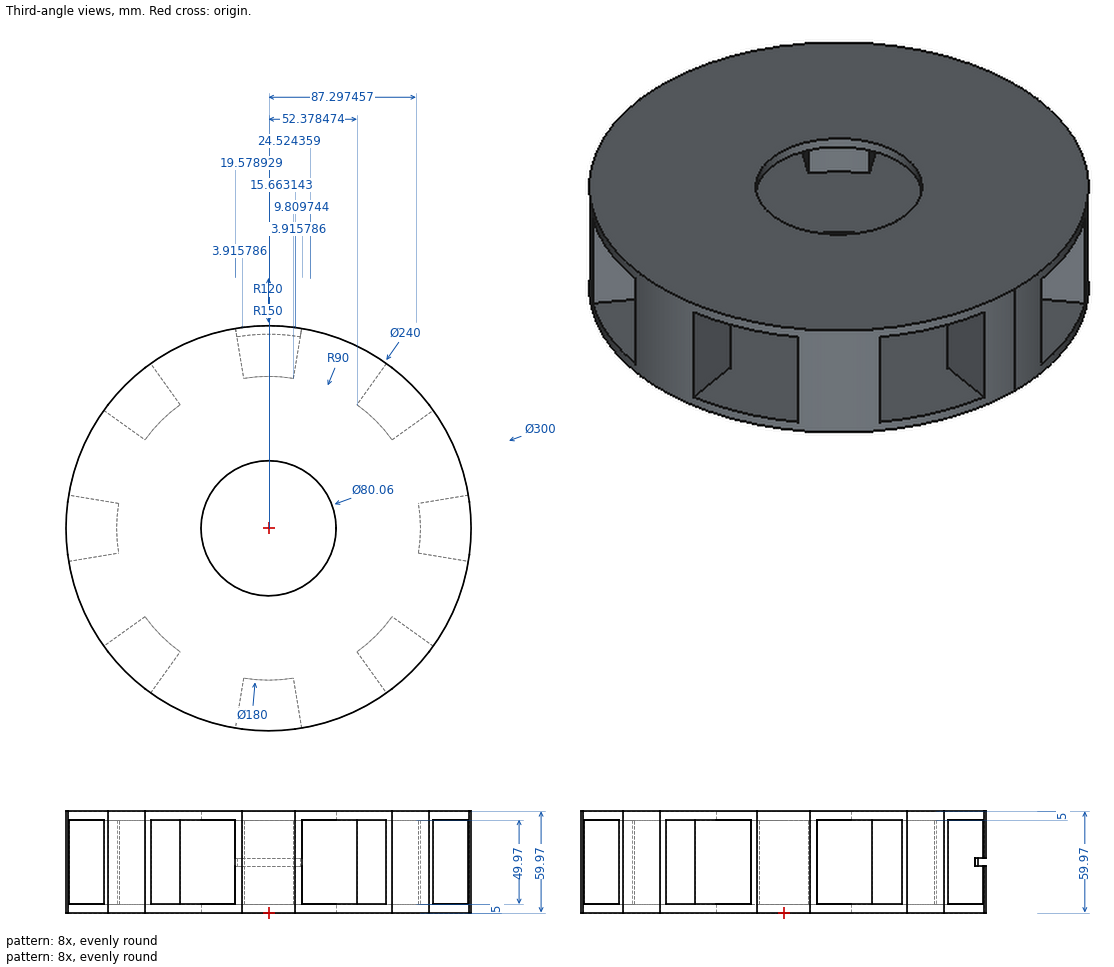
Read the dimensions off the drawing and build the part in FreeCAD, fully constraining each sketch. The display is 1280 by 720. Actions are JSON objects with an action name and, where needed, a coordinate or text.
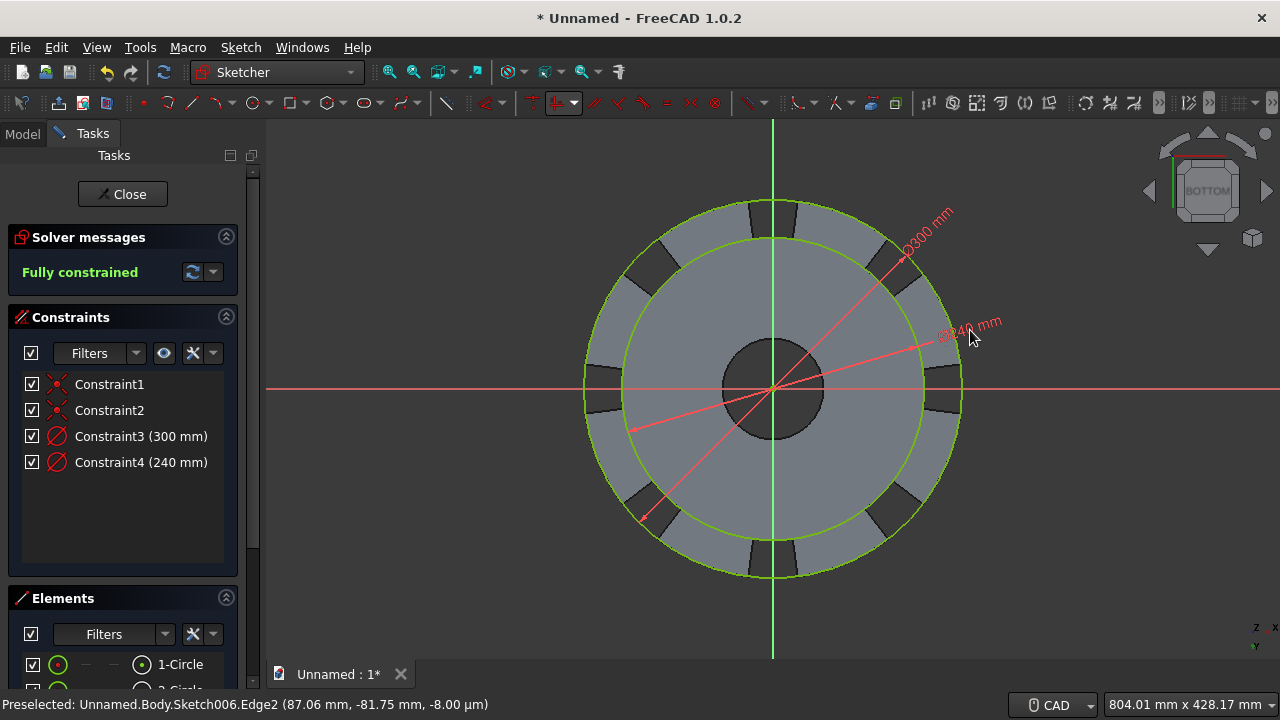
{"action": "left_click", "coordinate": [123, 194]}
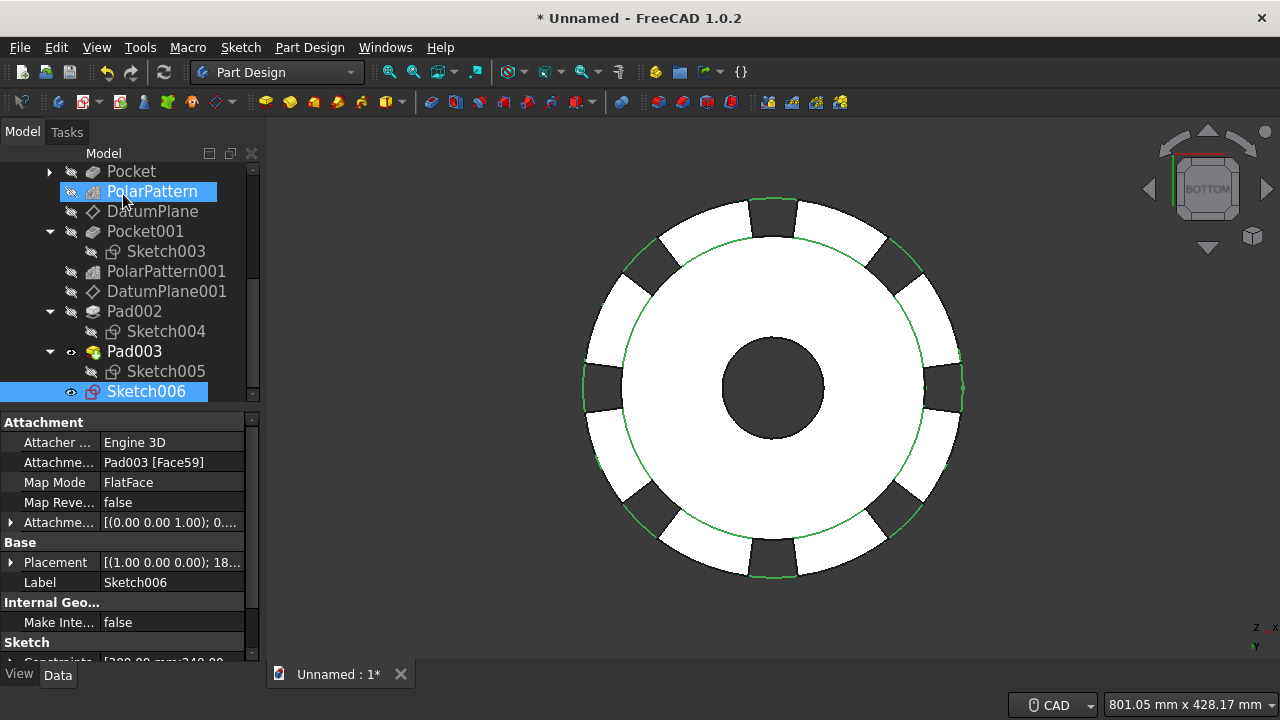
{"action": "left_click", "coordinate": [432, 102]}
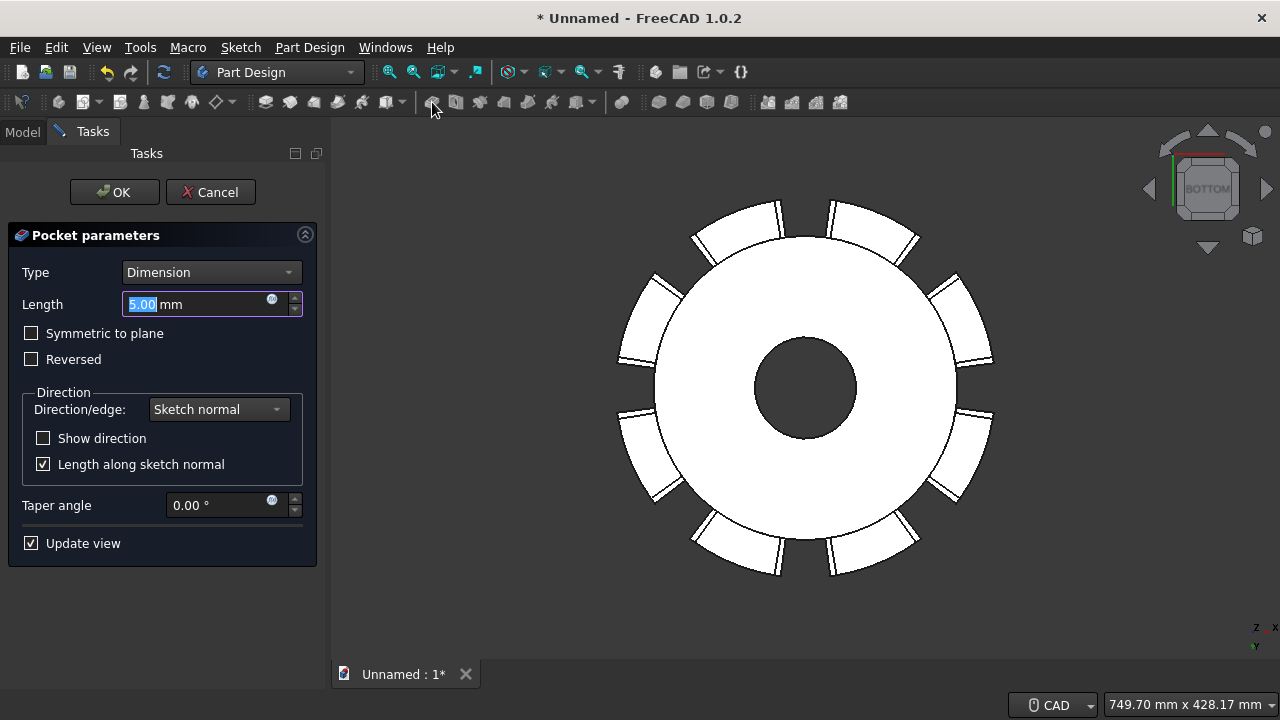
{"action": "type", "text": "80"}
{"action": "key", "text": "Tab"}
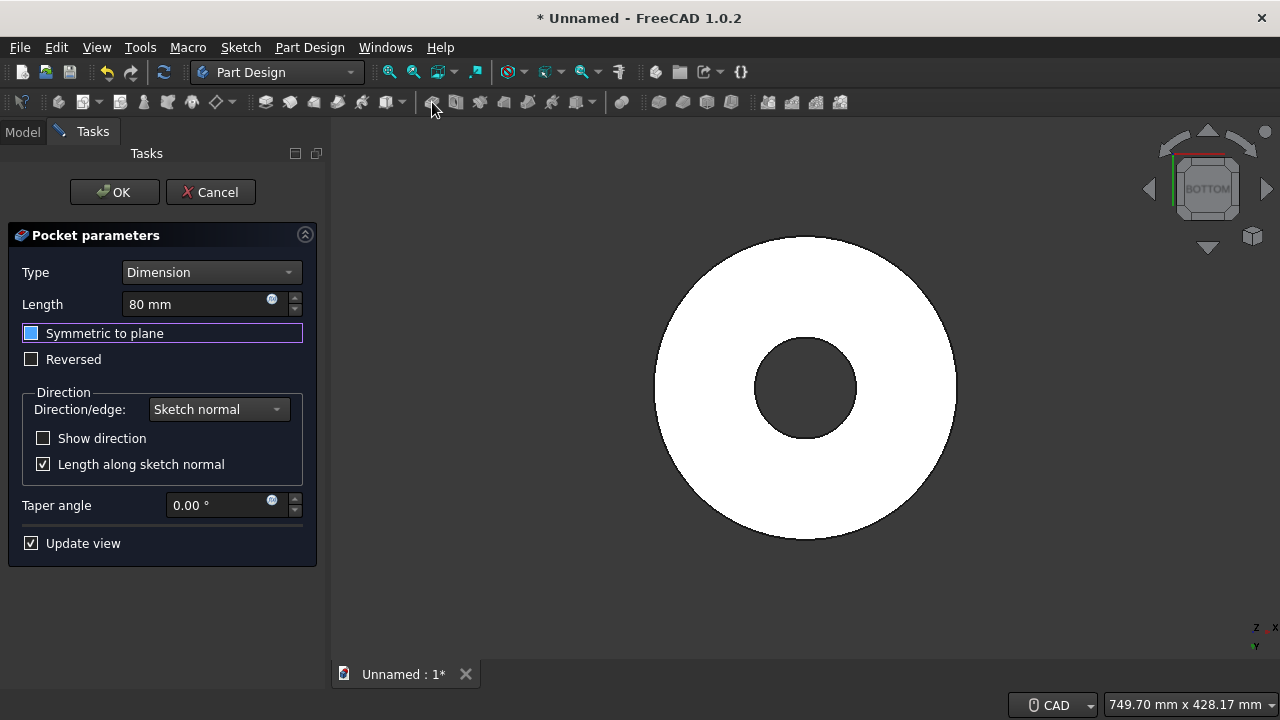
{"action": "left_click", "coordinate": [115, 192]}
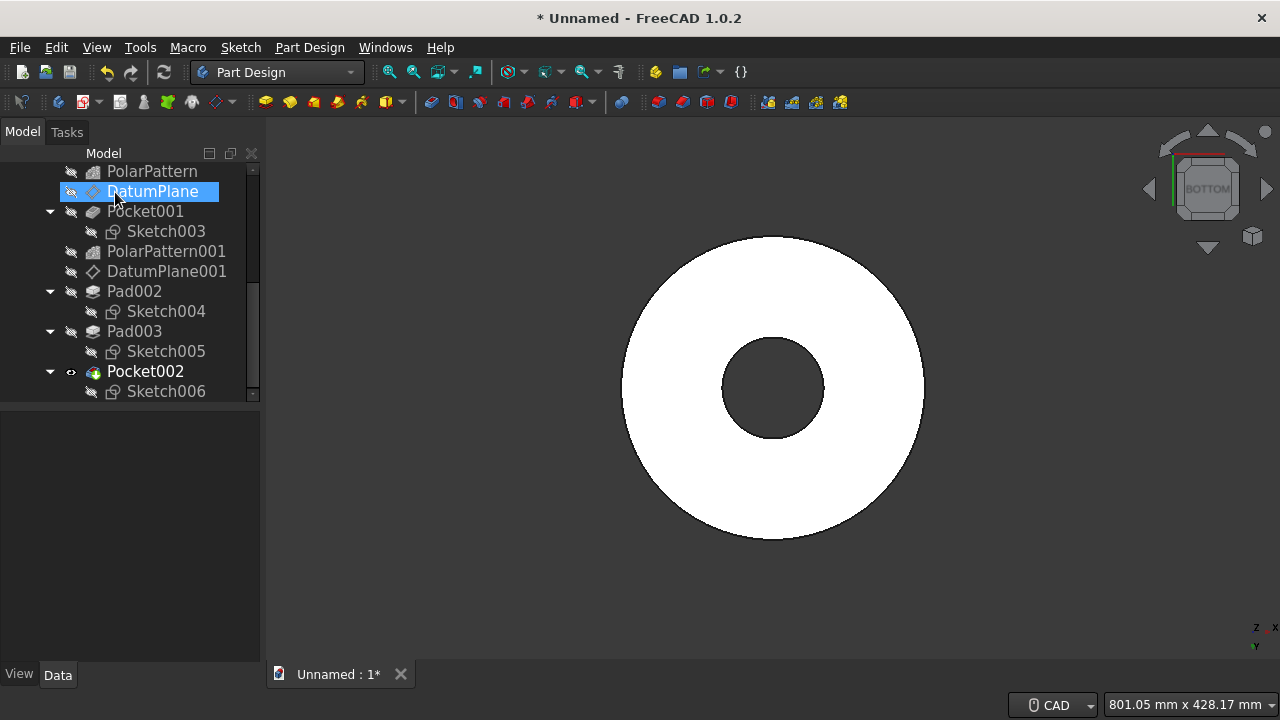
{"action": "key", "text": "6"}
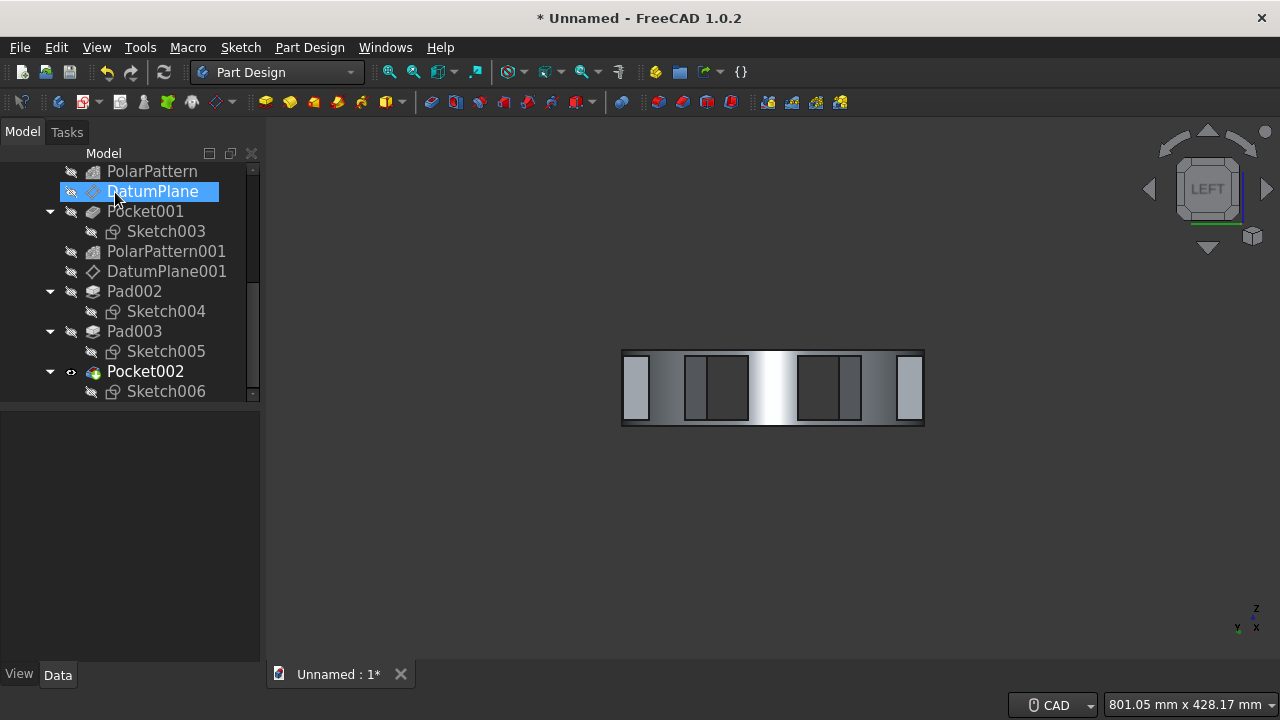
{"action": "left_click", "coordinate": [390, 72]}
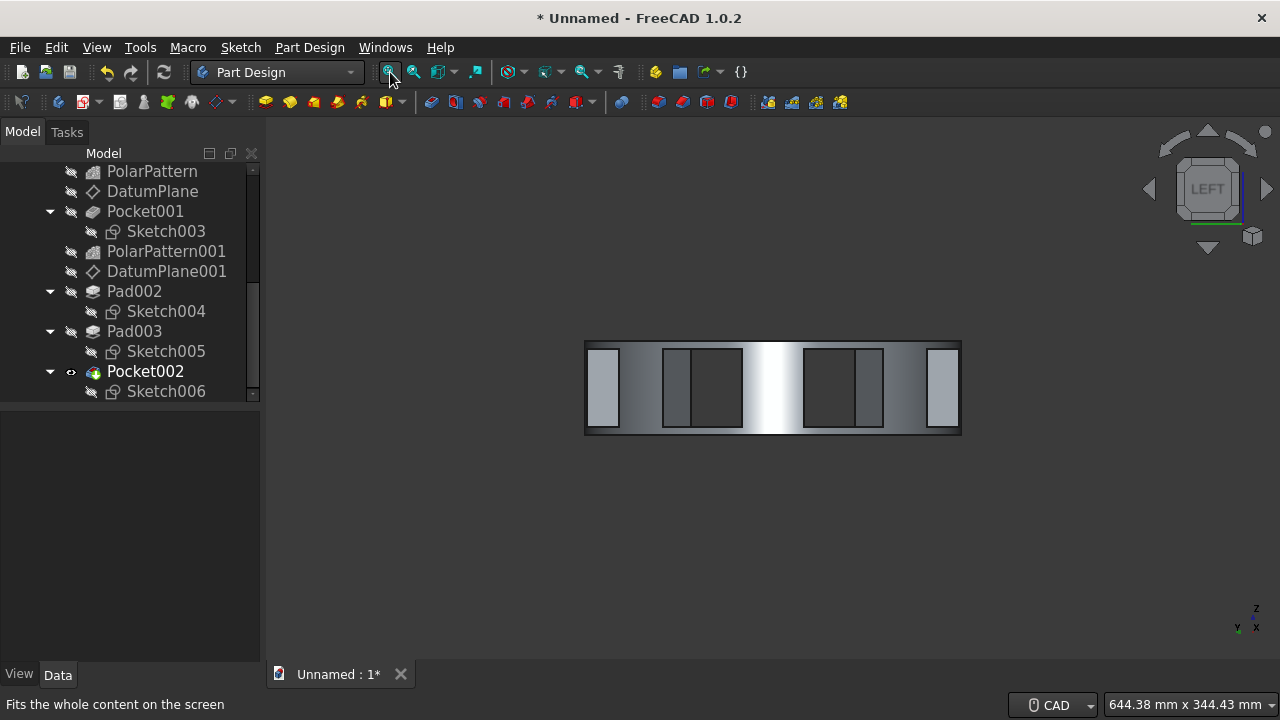
{"action": "left_click", "coordinate": [943, 376]}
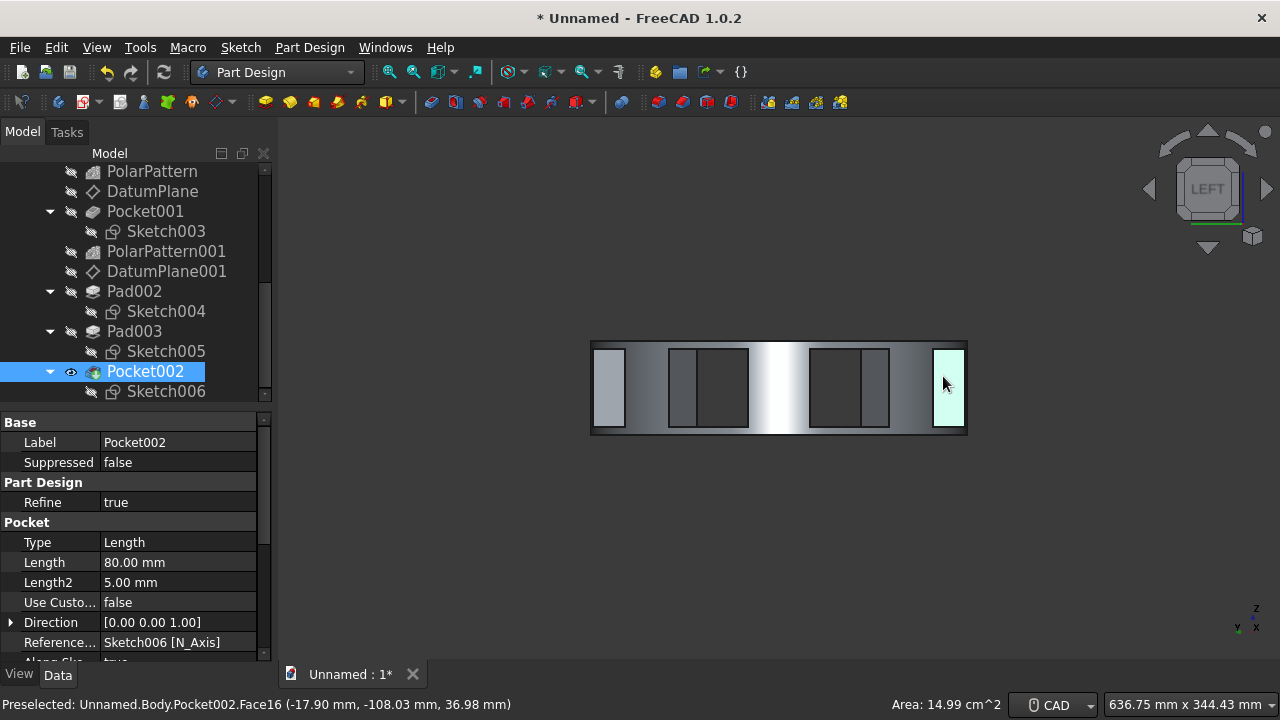
{"action": "left_click", "coordinate": [84, 102]}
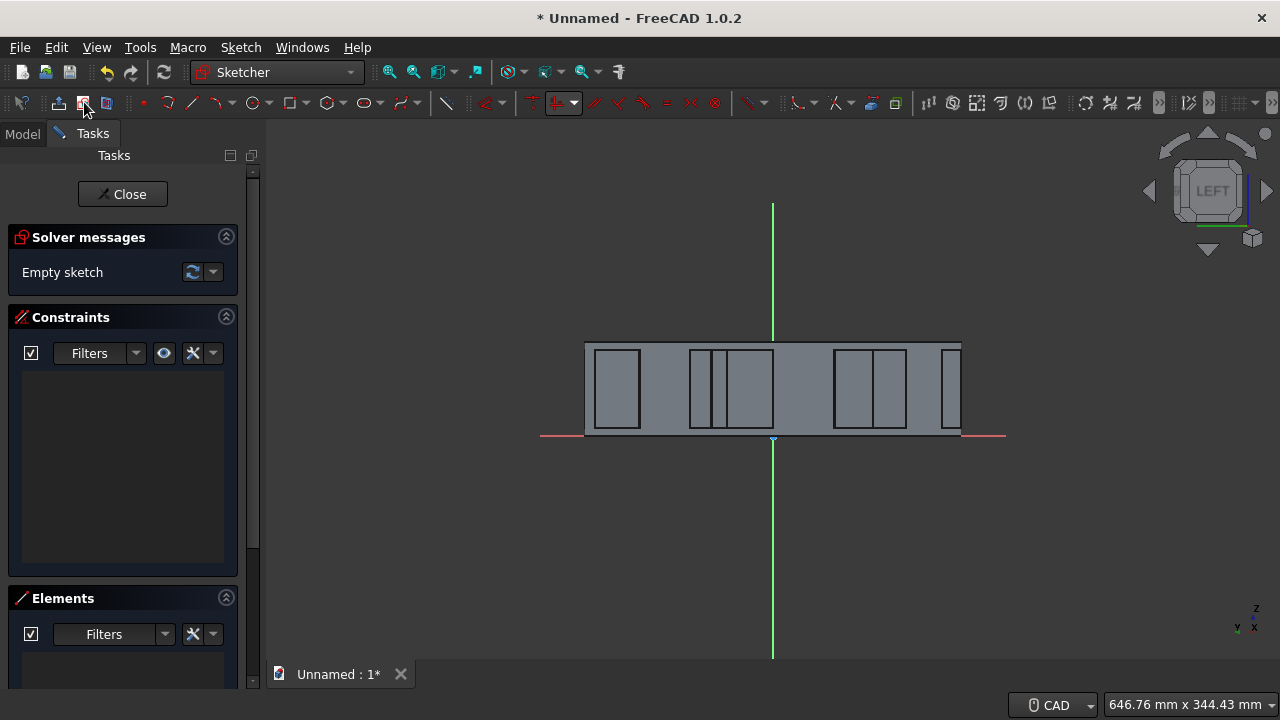
{"action": "scroll", "coordinate": [583, 389], "scroll_direction": "up", "scroll_amount": 15}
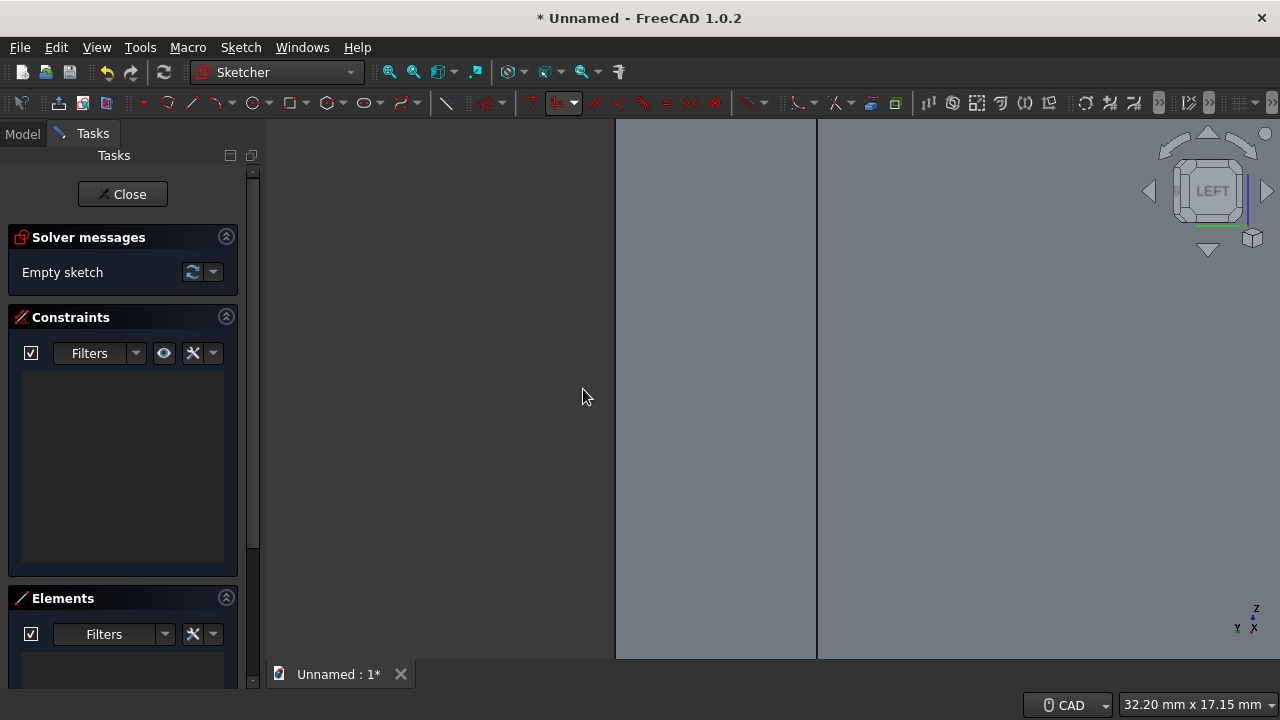
{"action": "scroll", "coordinate": [684, 372], "scroll_direction": "up", "scroll_amount": 4}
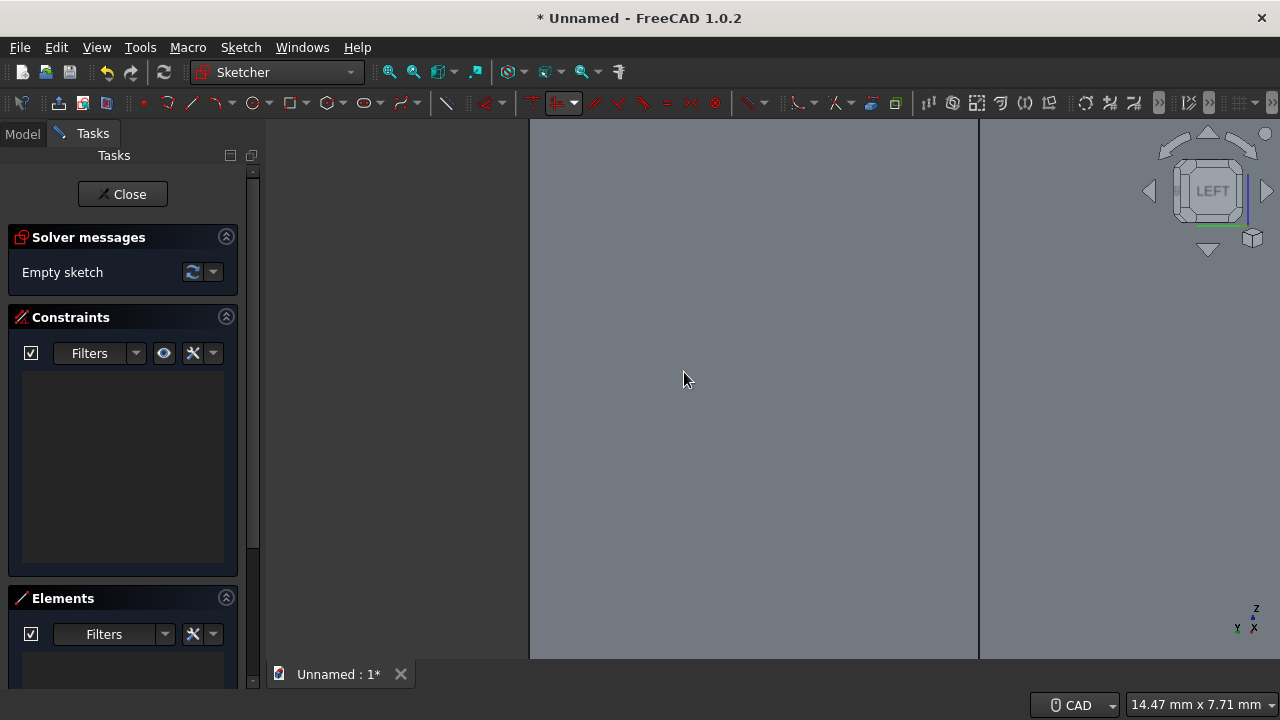
{"action": "left_click", "coordinate": [290, 104]}